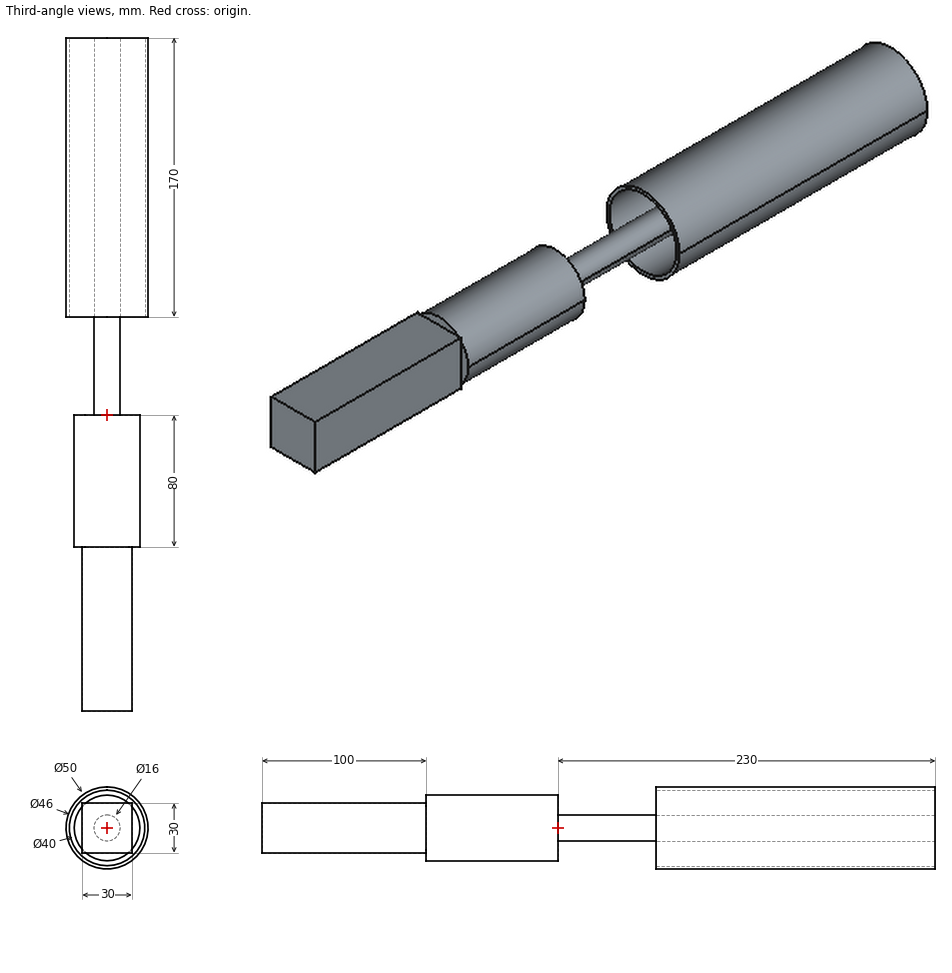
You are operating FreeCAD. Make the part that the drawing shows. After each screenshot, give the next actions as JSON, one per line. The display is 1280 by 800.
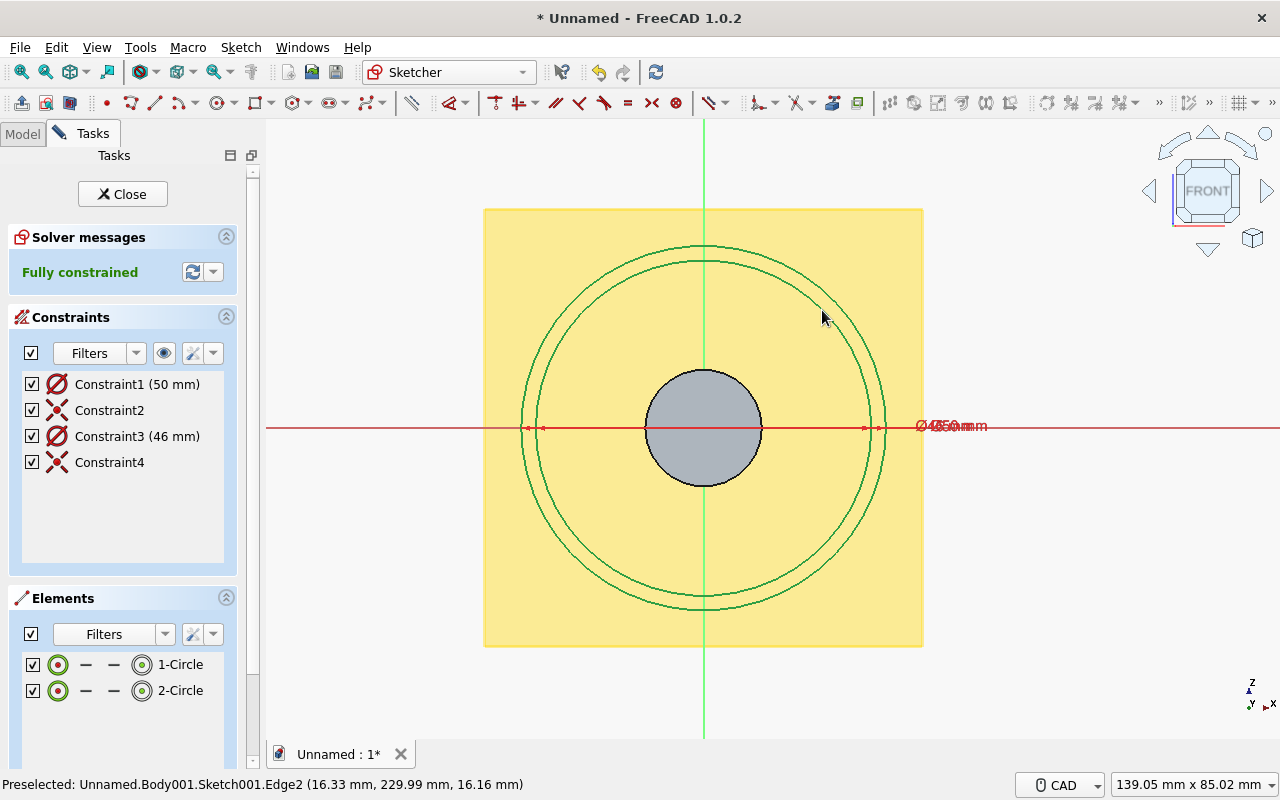
{"action": "left_click", "coordinate": [123, 194]}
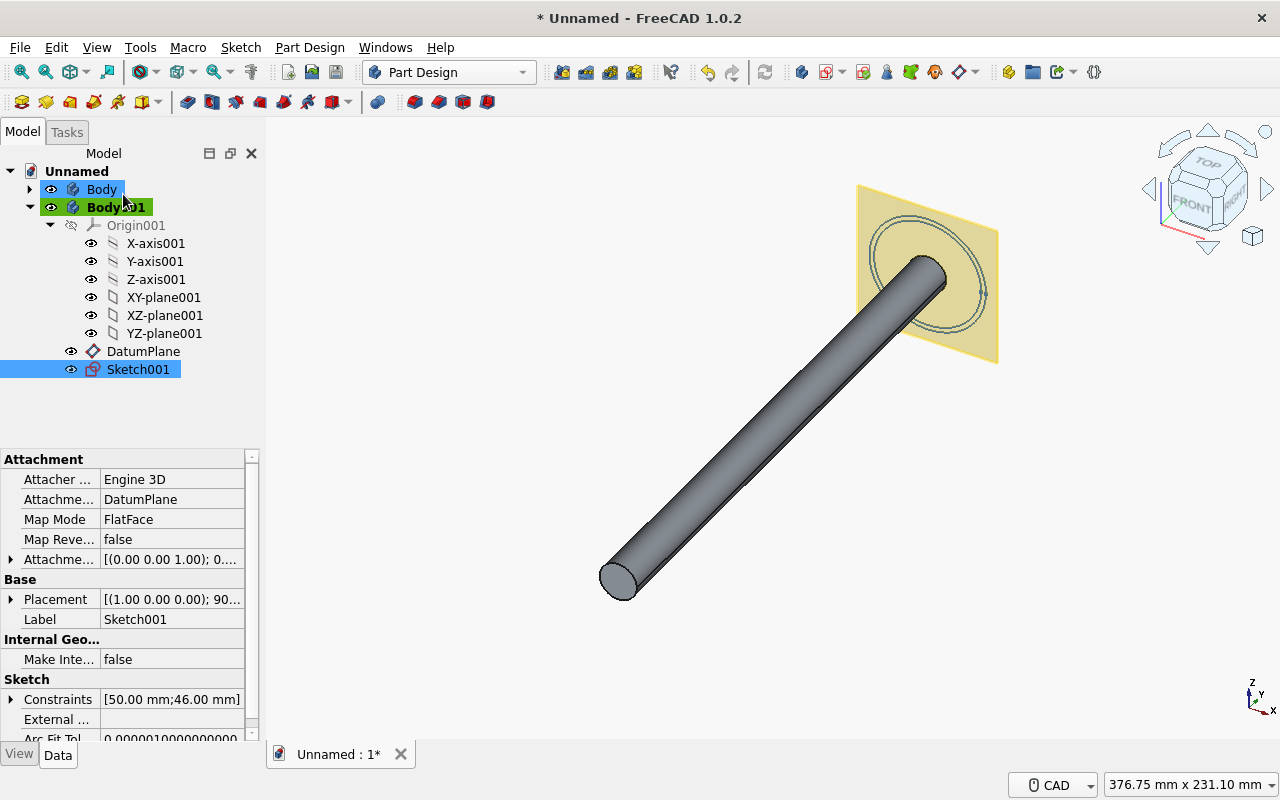
{"action": "left_click", "coordinate": [22, 102]}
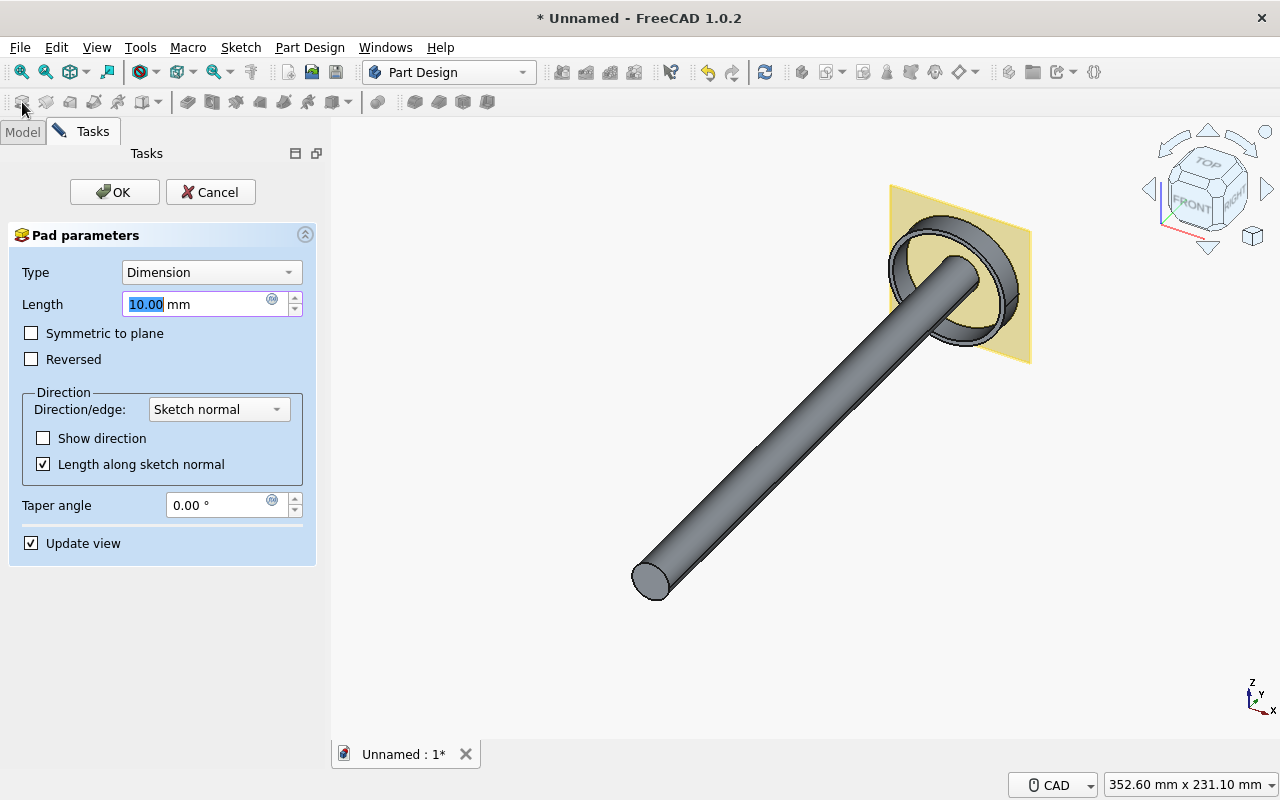
{"action": "type", "text": "170"}
{"action": "key", "text": "Tab"}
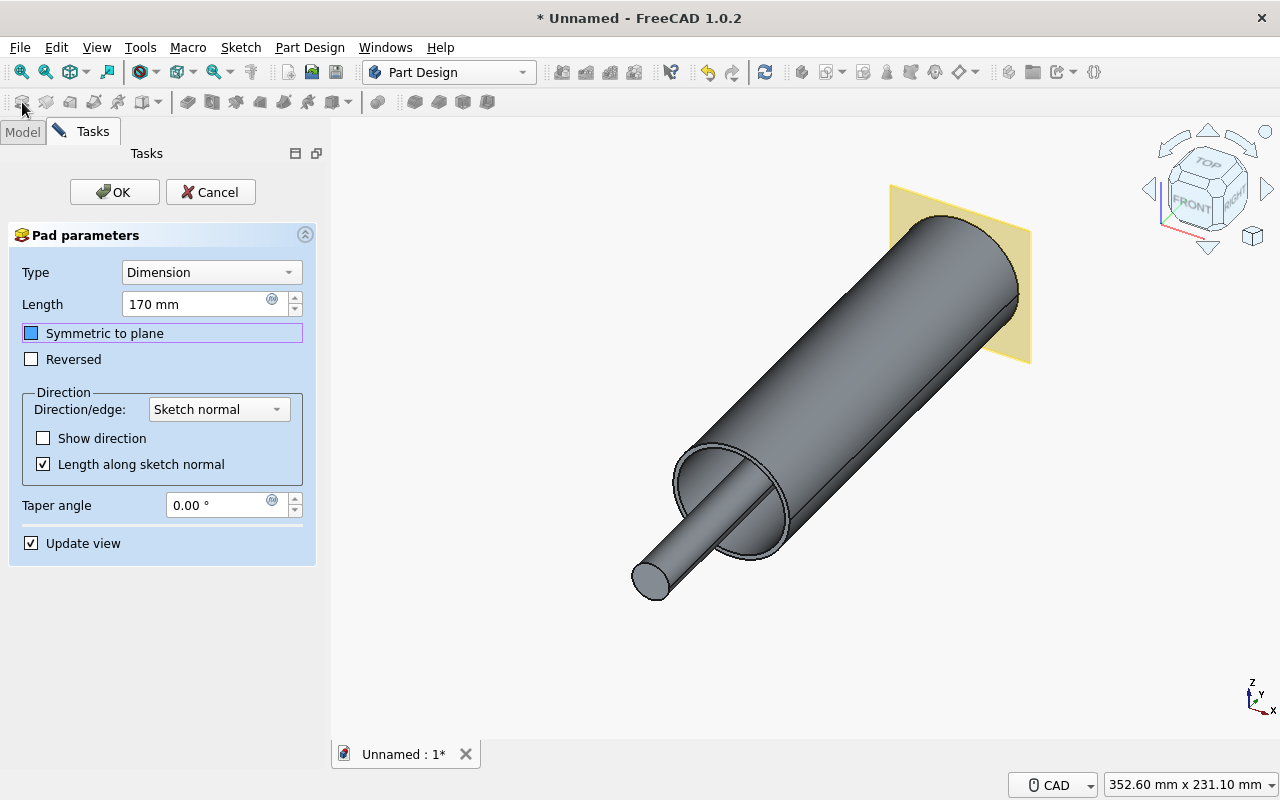
{"action": "left_click", "coordinate": [115, 192]}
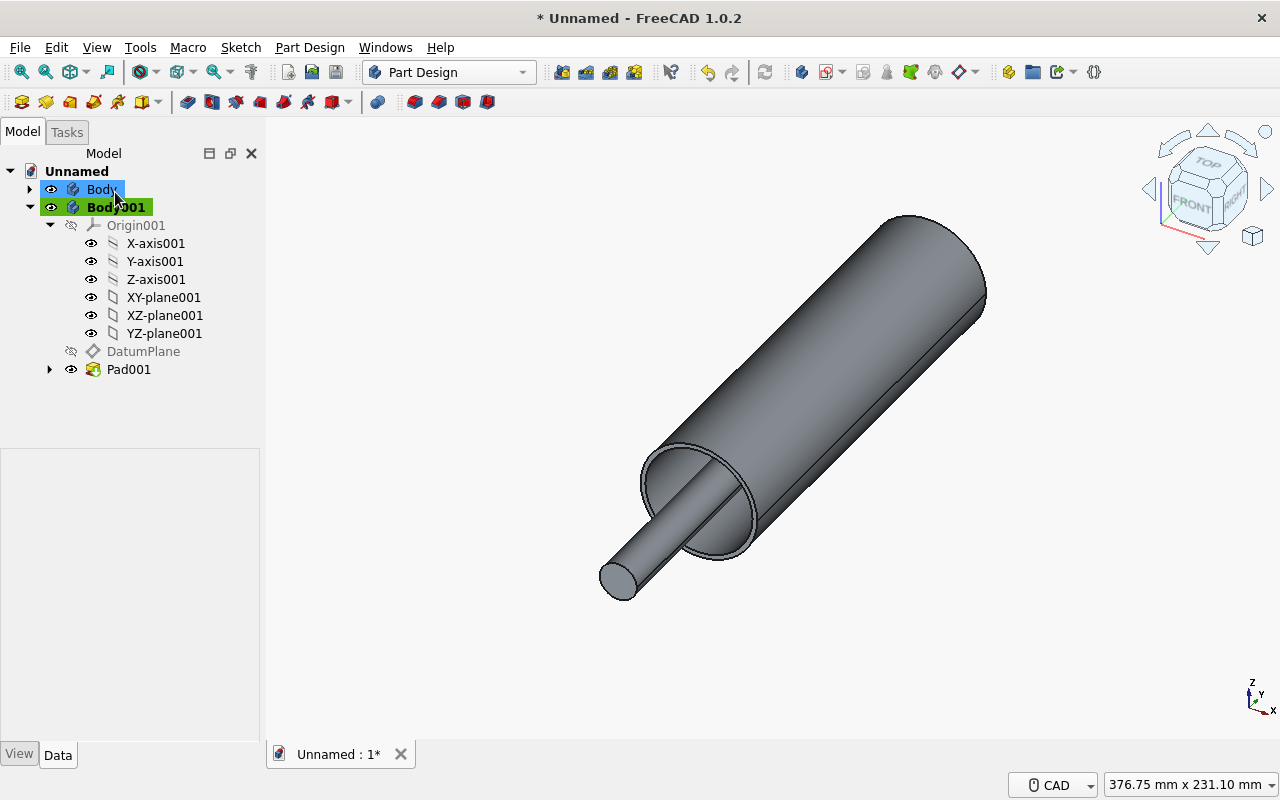
{"action": "left_click", "coordinate": [802, 72]}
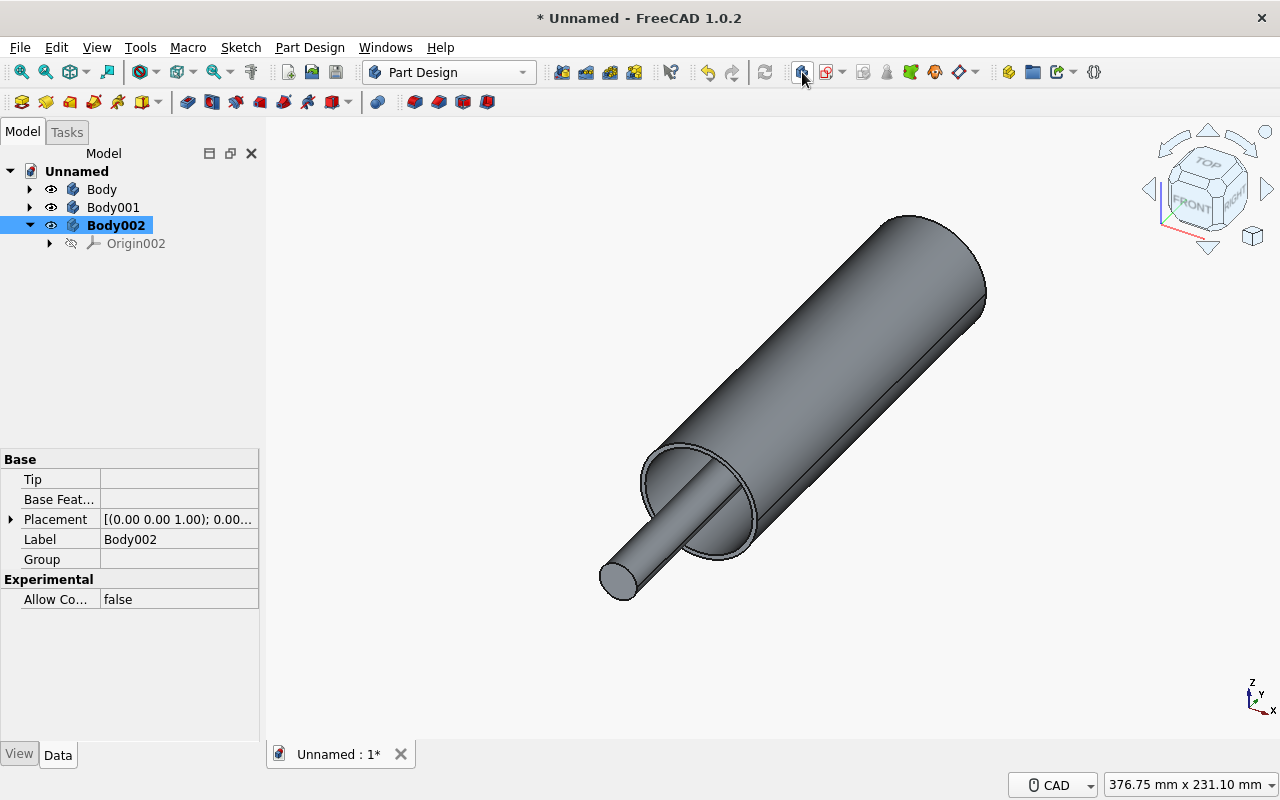
{"action": "left_click", "coordinate": [50, 243]}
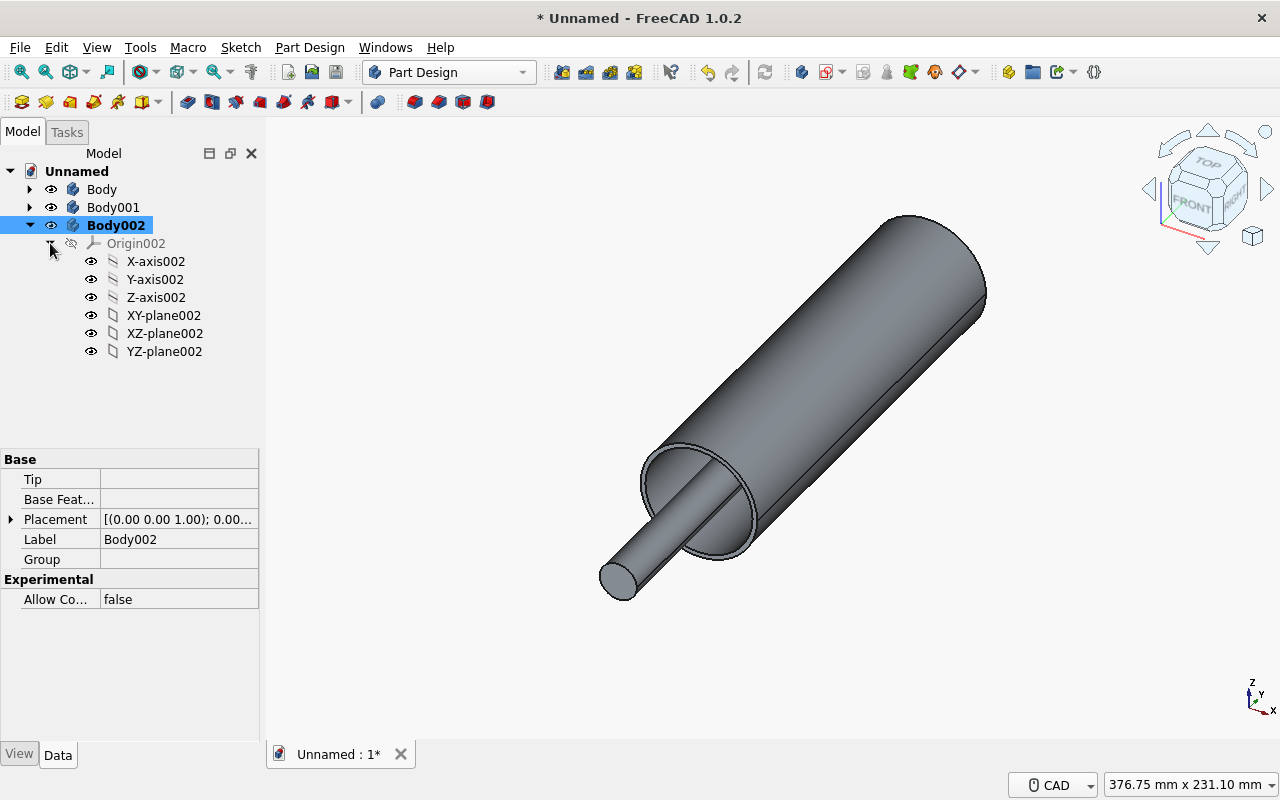
{"action": "left_click", "coordinate": [136, 333]}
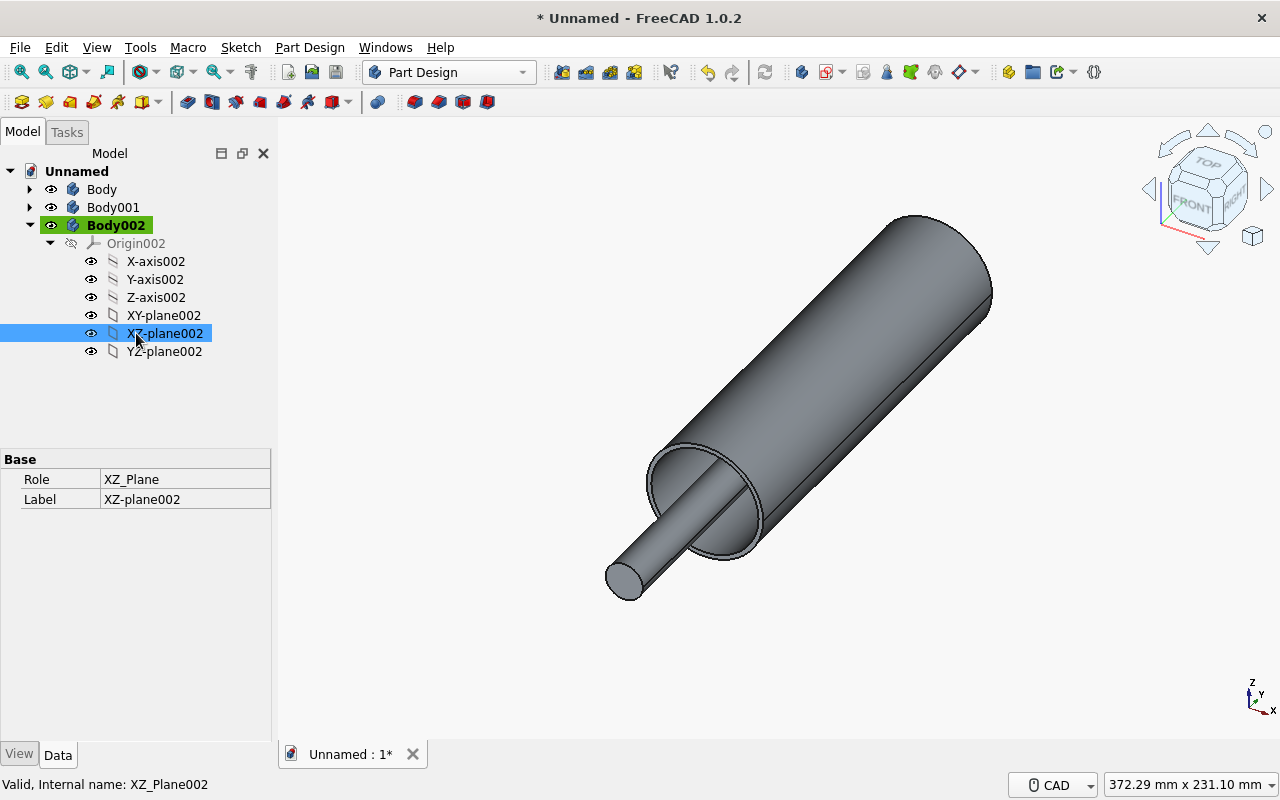
{"action": "left_click", "coordinate": [960, 72]}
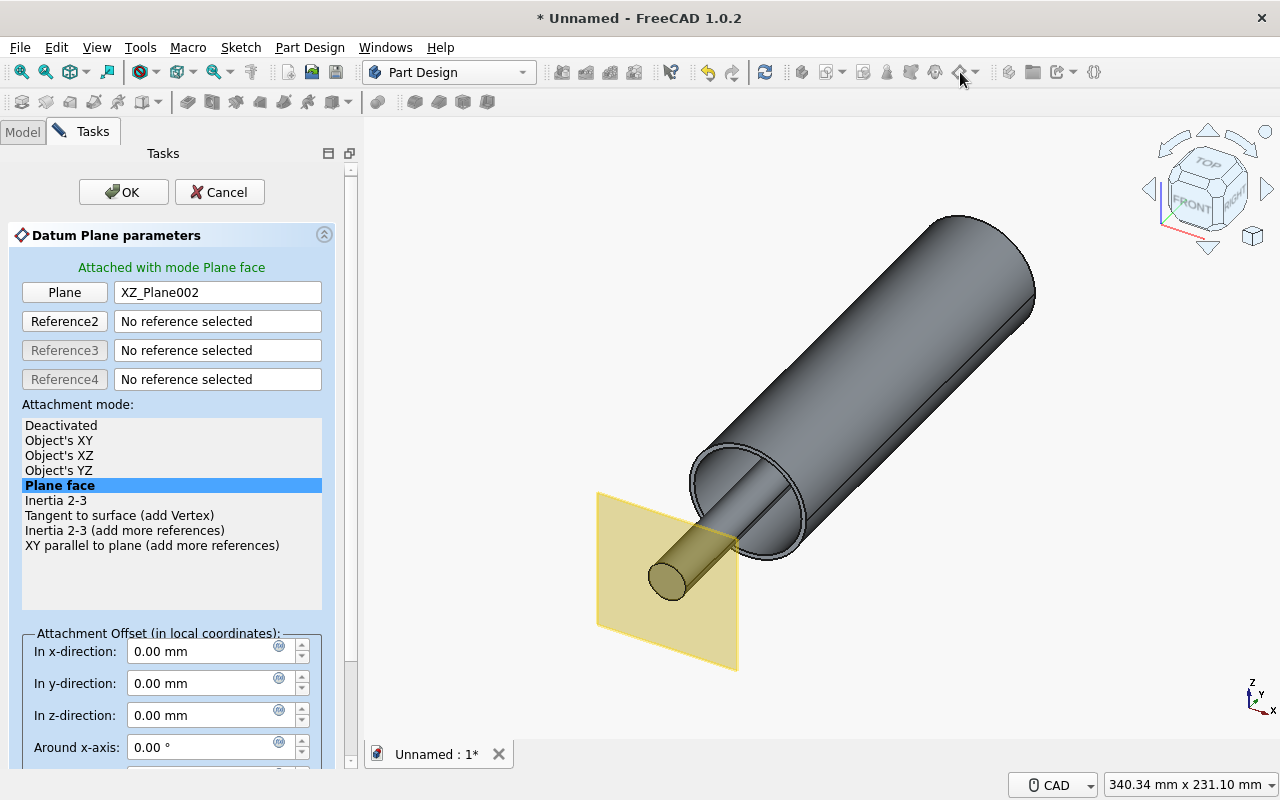
{"action": "triple_click", "coordinate": [210, 715]}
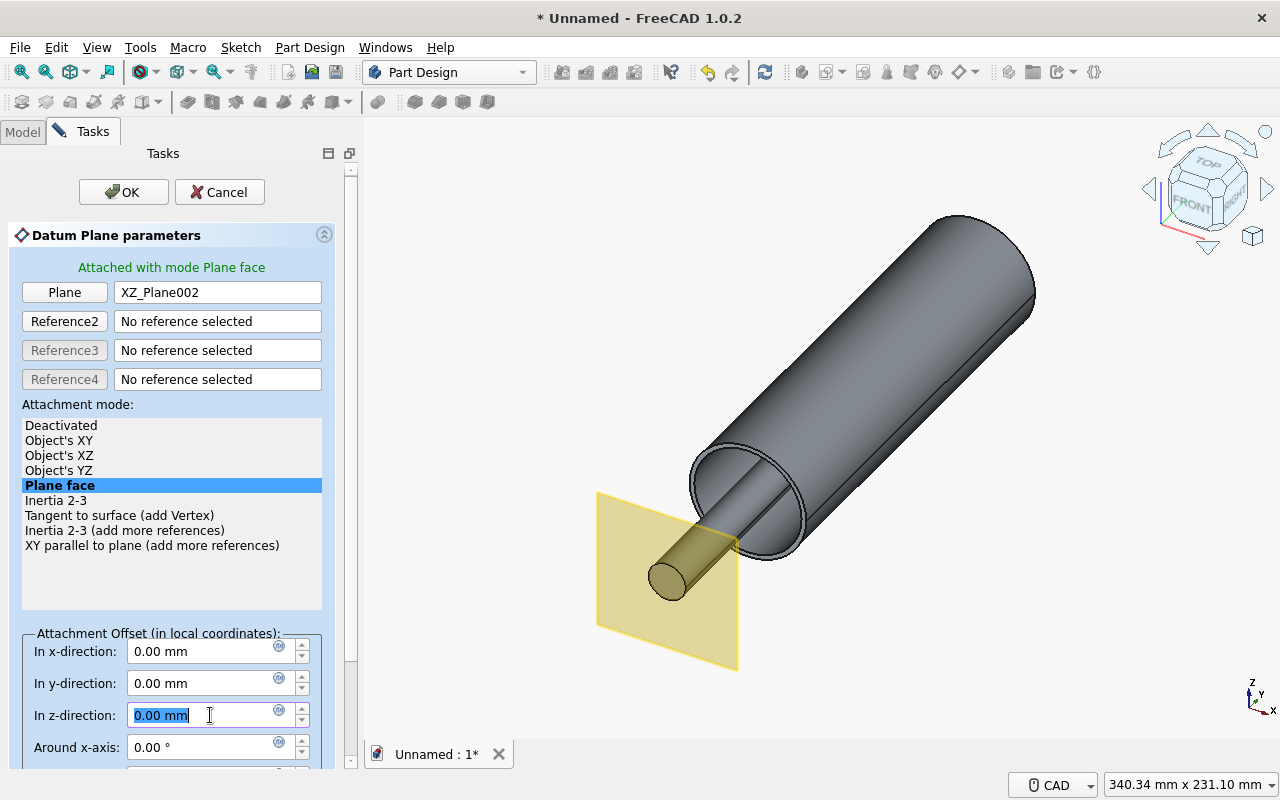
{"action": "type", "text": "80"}
{"action": "key", "text": "Tab"}